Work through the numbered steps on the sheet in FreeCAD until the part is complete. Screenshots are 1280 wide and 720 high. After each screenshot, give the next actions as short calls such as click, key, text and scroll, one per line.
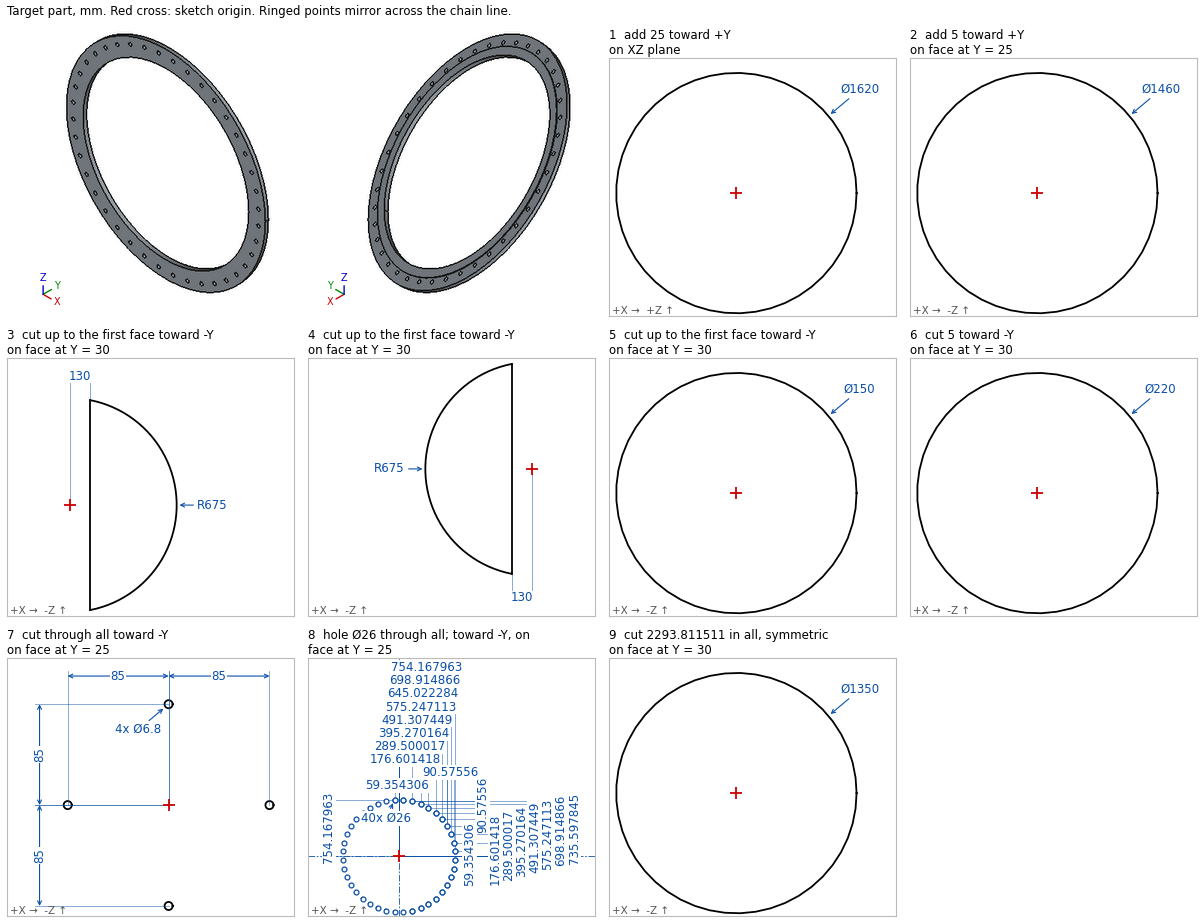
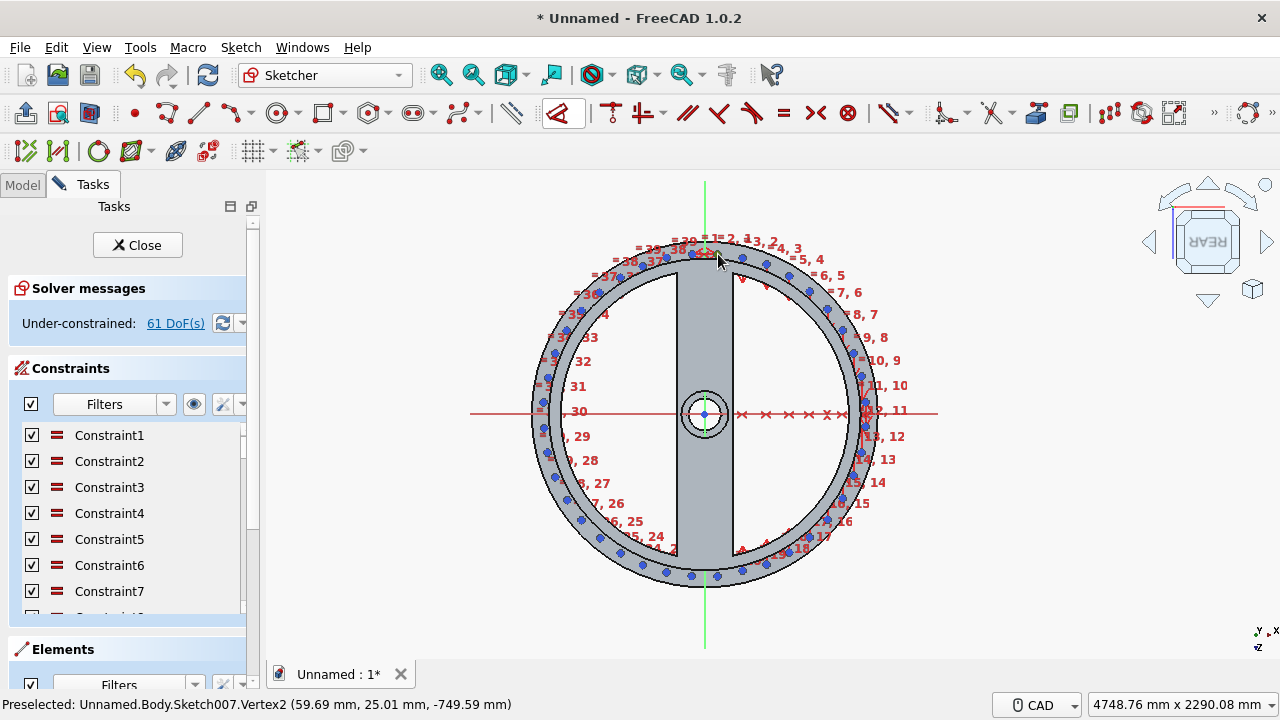
click(718, 576)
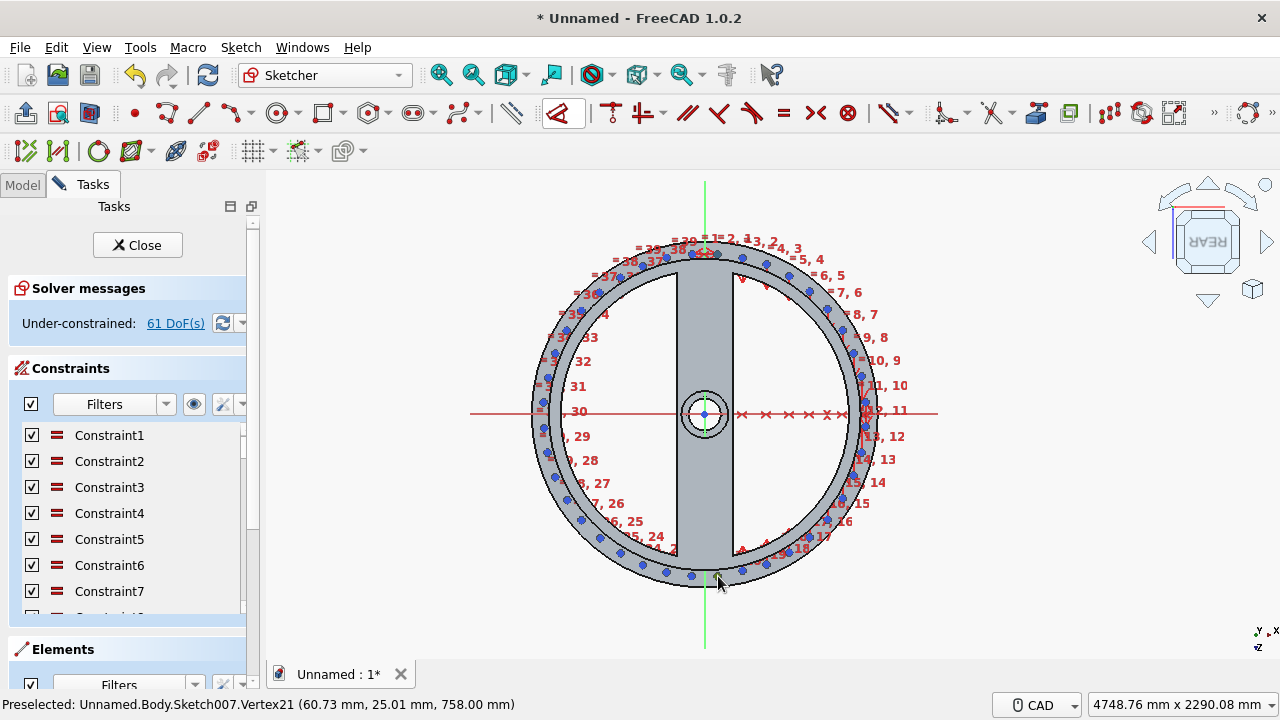
click(470, 414)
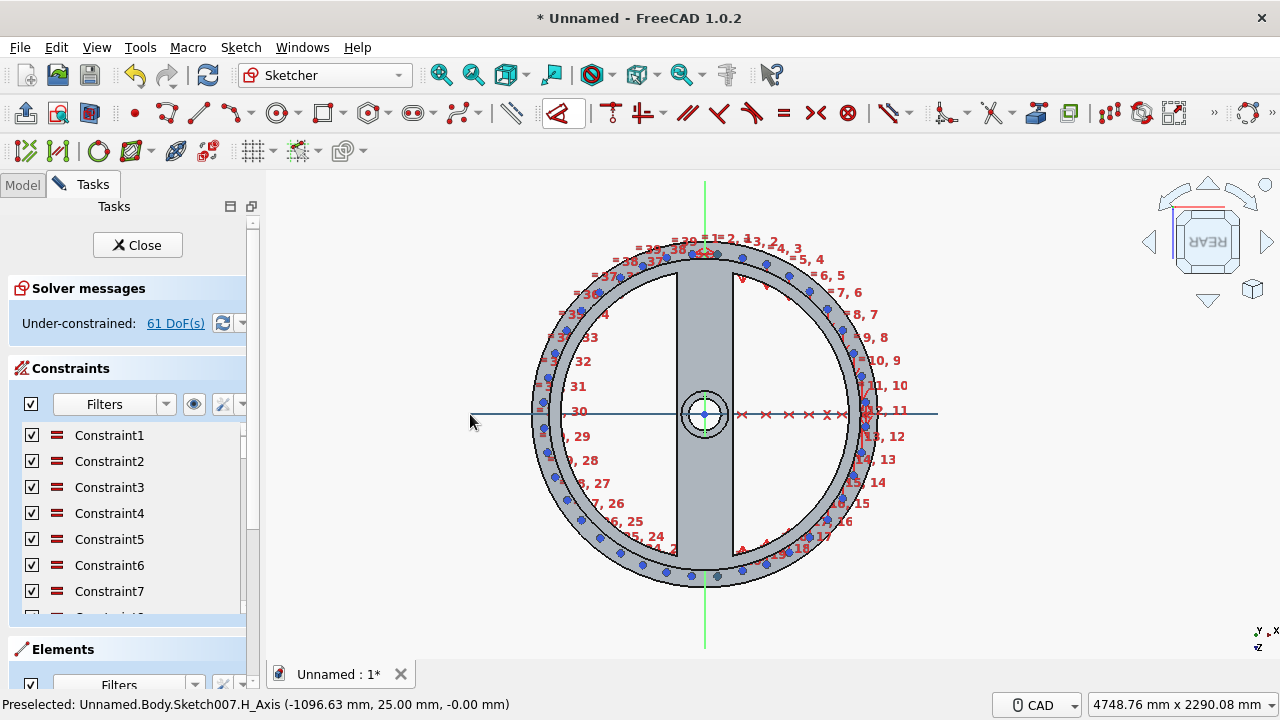
key(s)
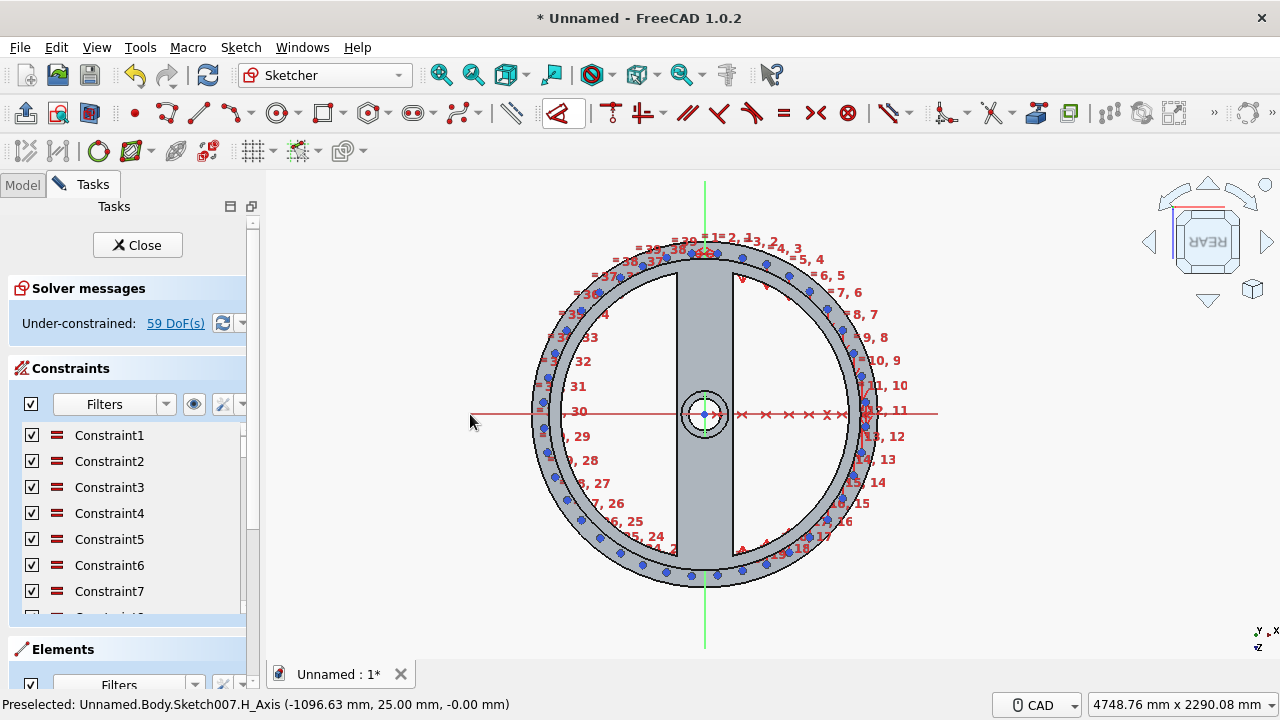
click(692, 254)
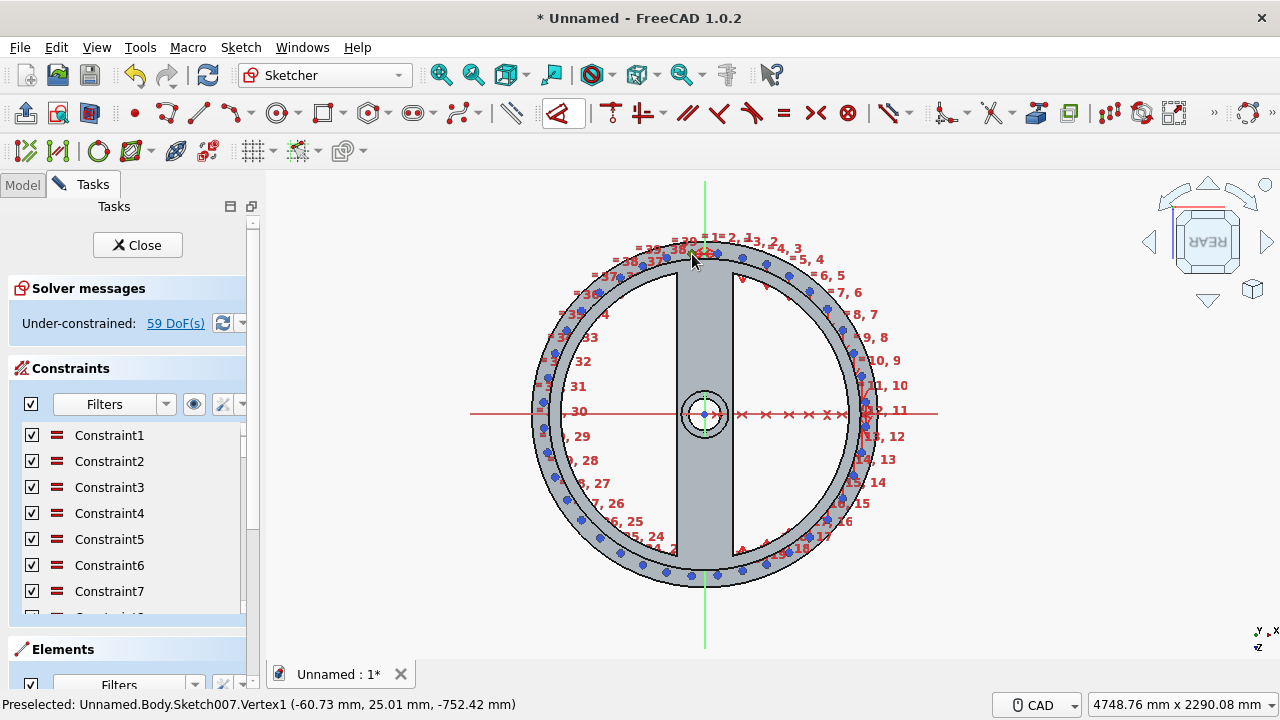
click(692, 576)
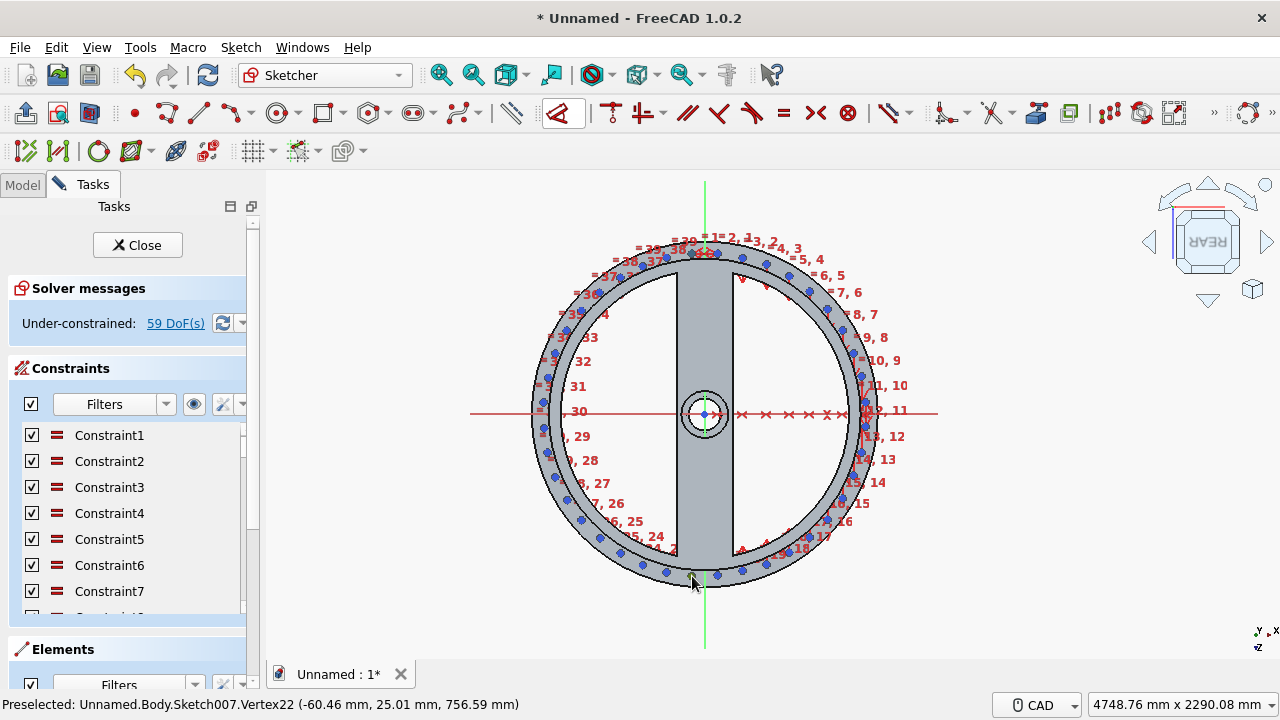
click(470, 414)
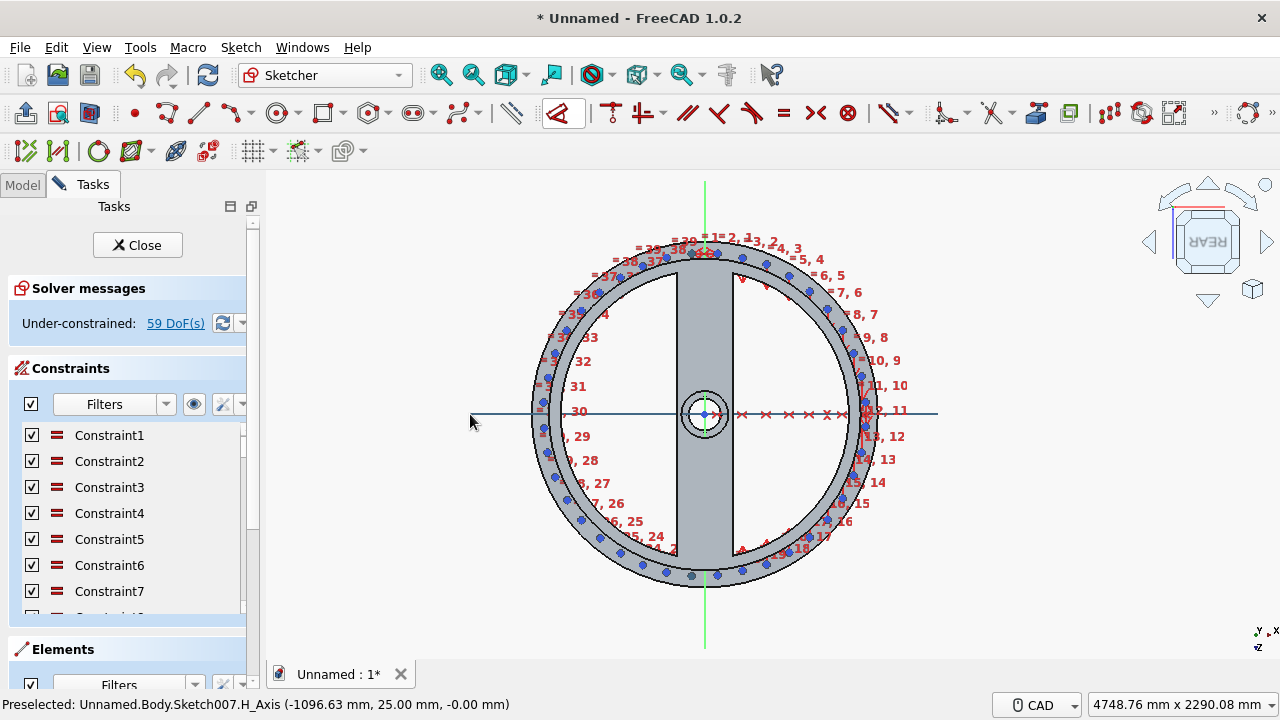
click(816, 114)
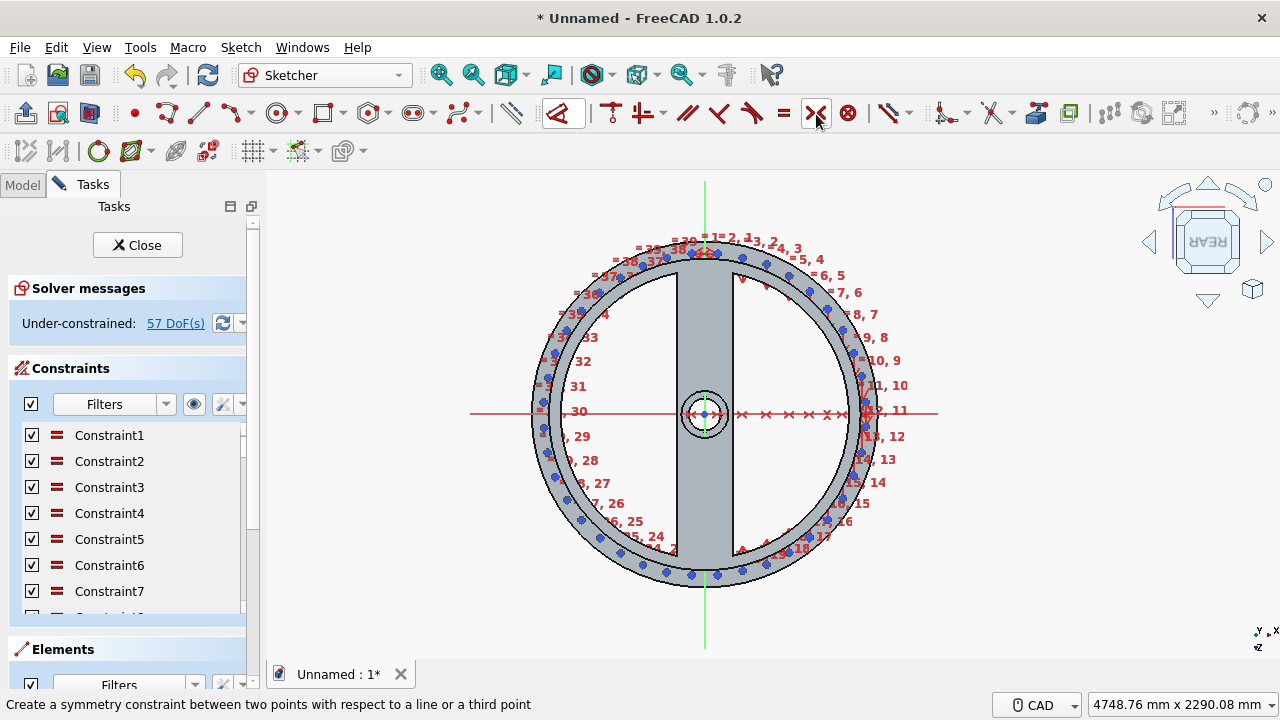
click(743, 571)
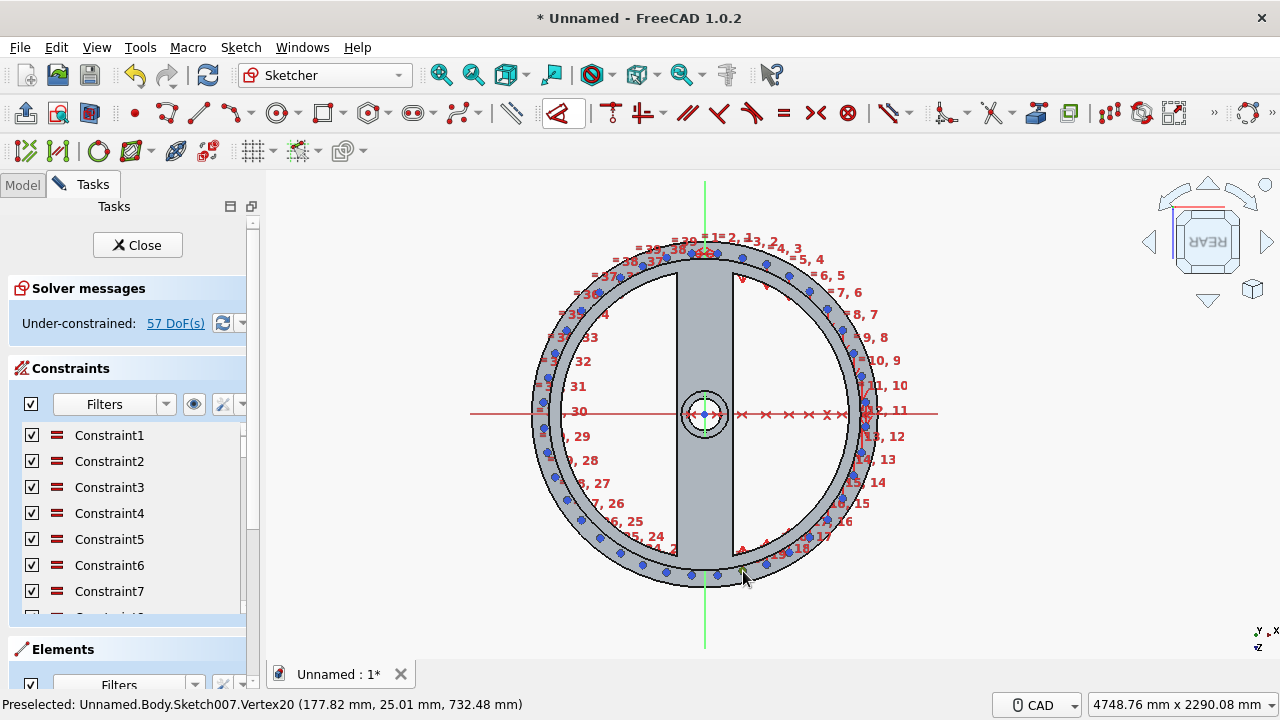
click(667, 572)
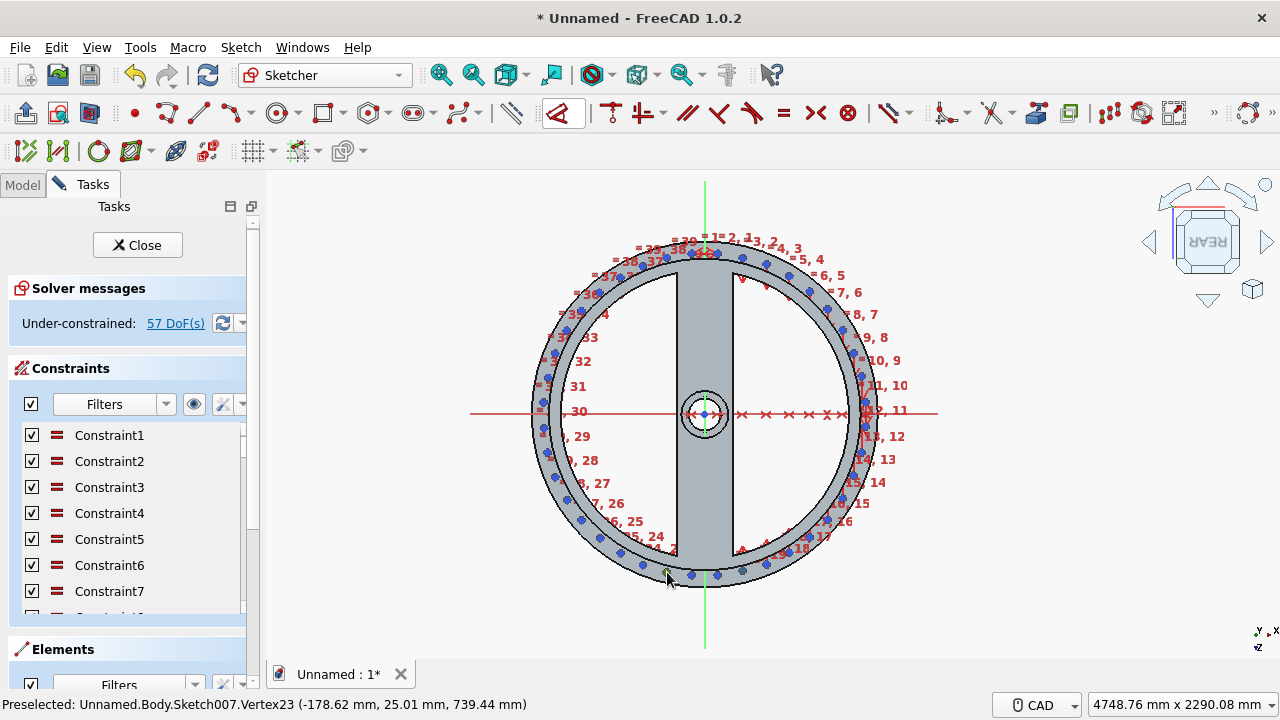
click(705, 538)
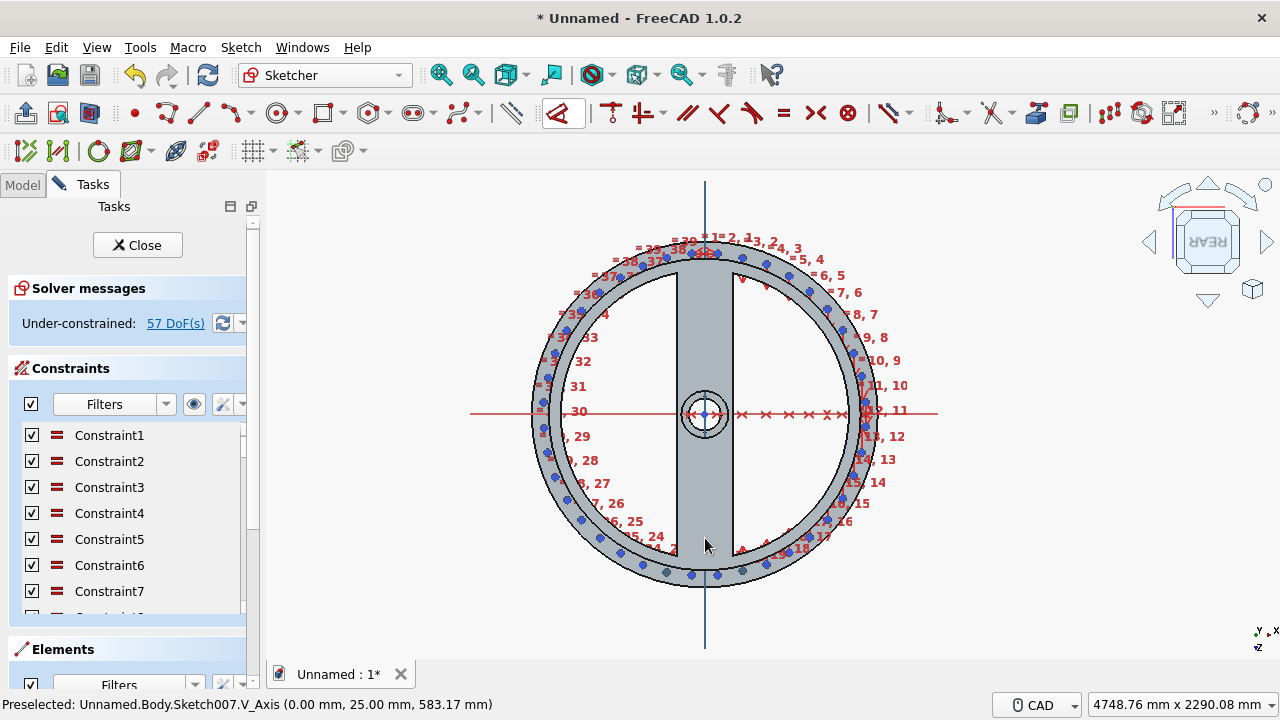
click(816, 114)